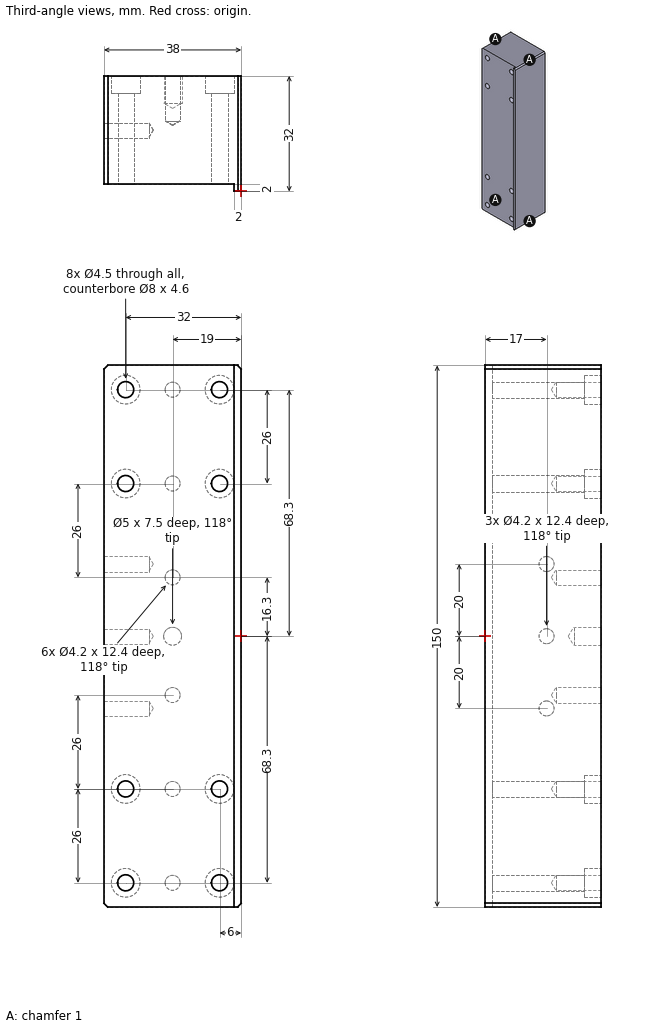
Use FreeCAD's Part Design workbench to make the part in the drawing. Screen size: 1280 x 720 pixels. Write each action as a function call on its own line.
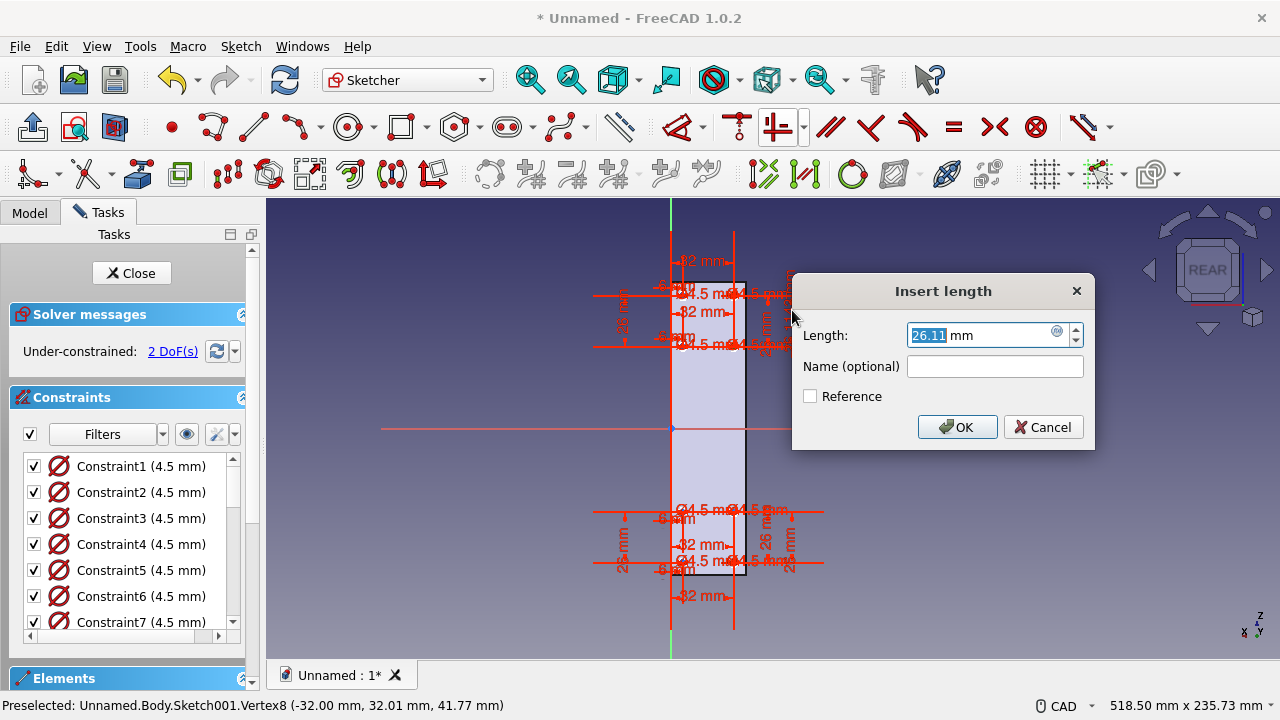
text(26)
key(Return)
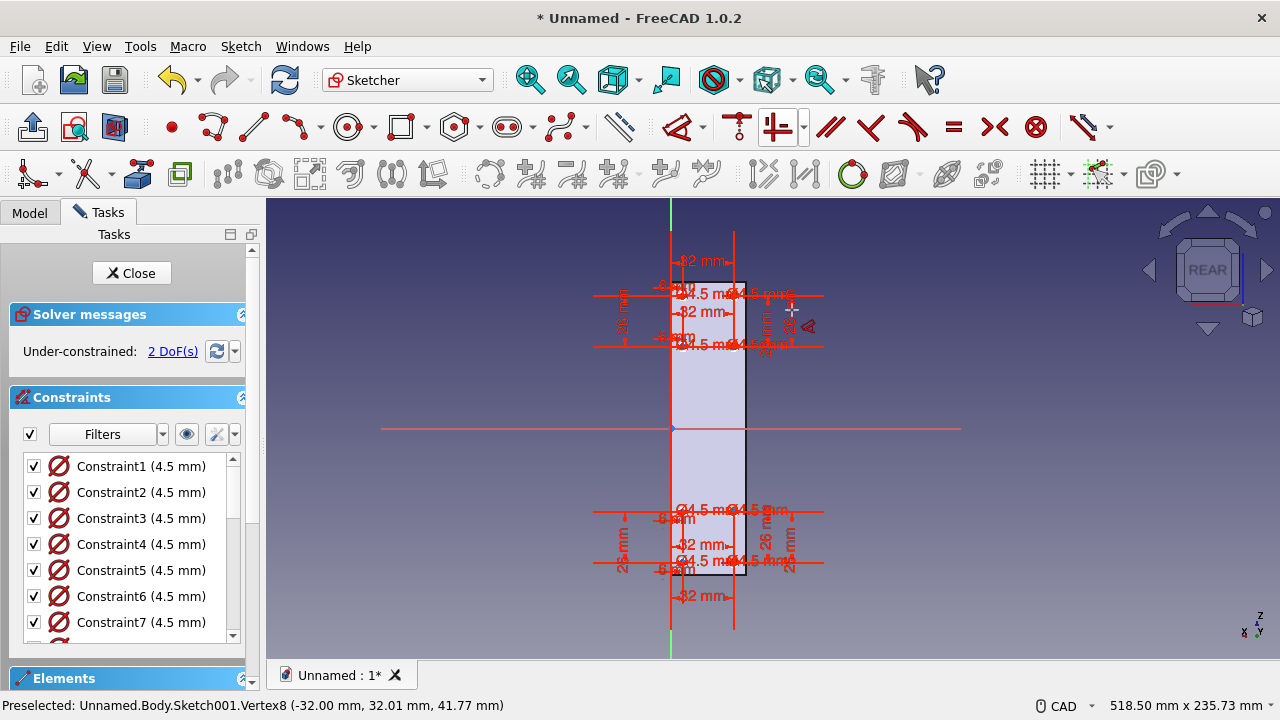
click(734, 296)
click(637, 362)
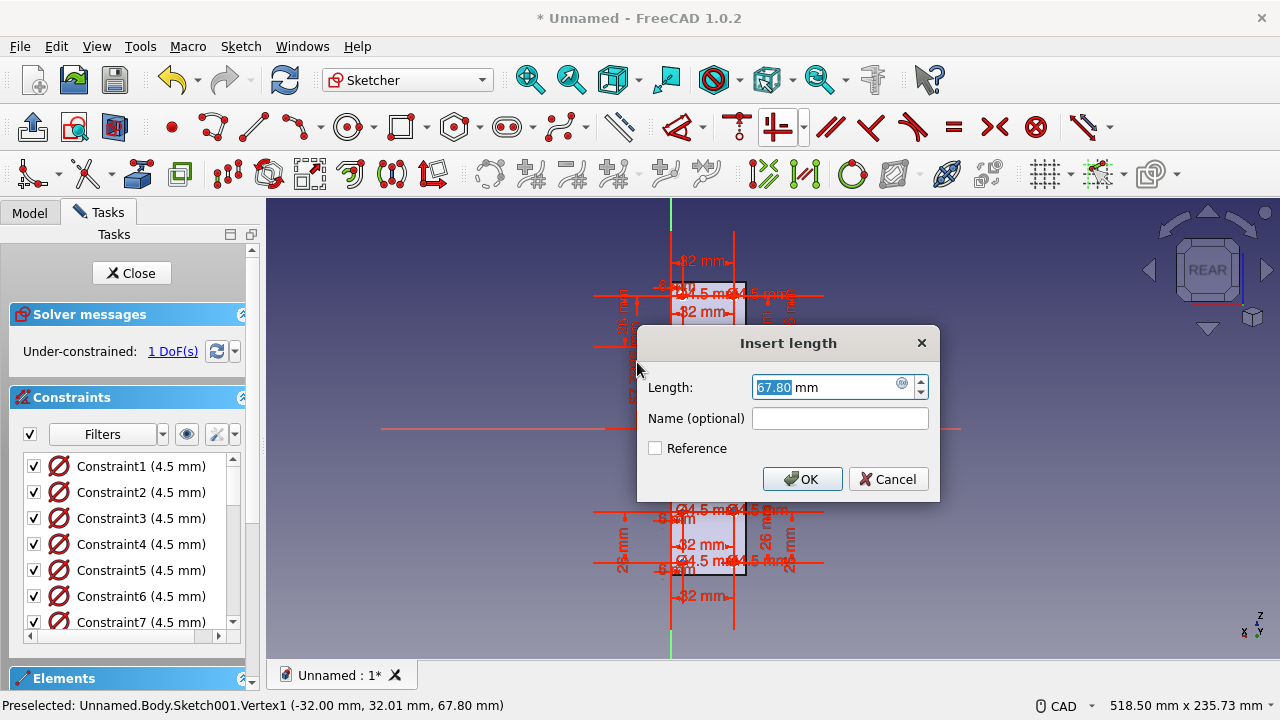
text(68.3)
key(Return)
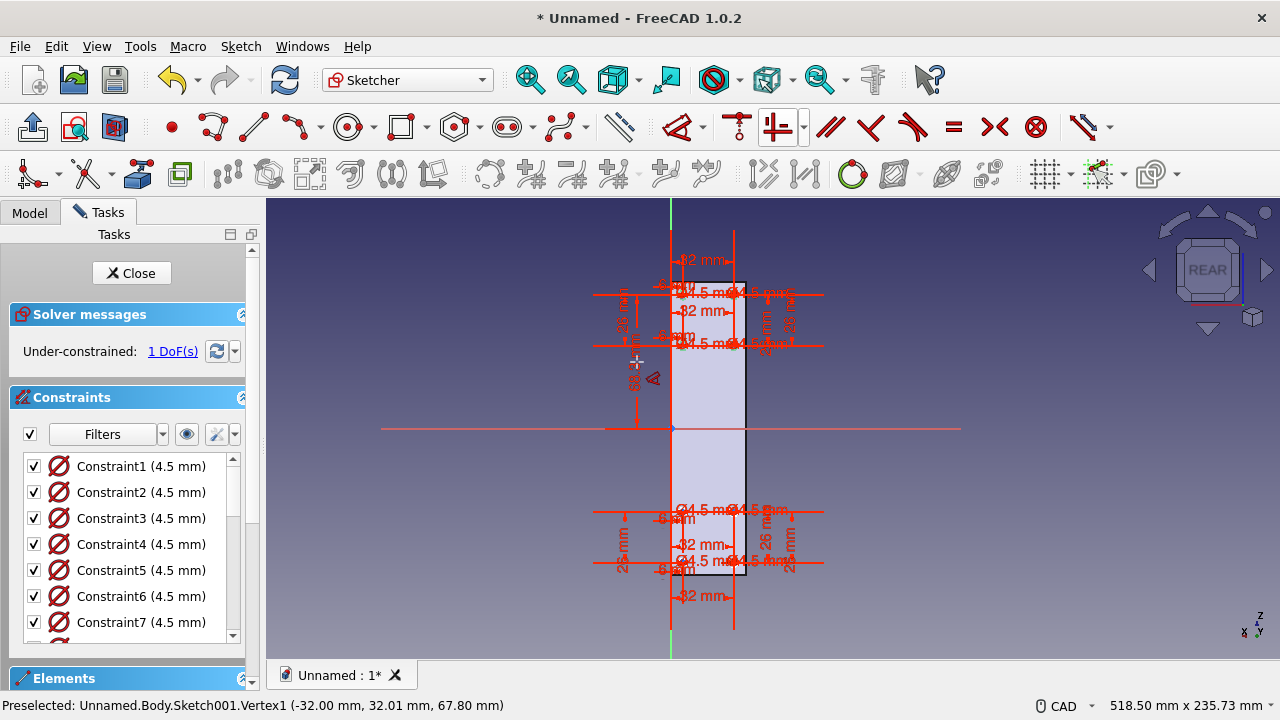
click(734, 563)
click(637, 496)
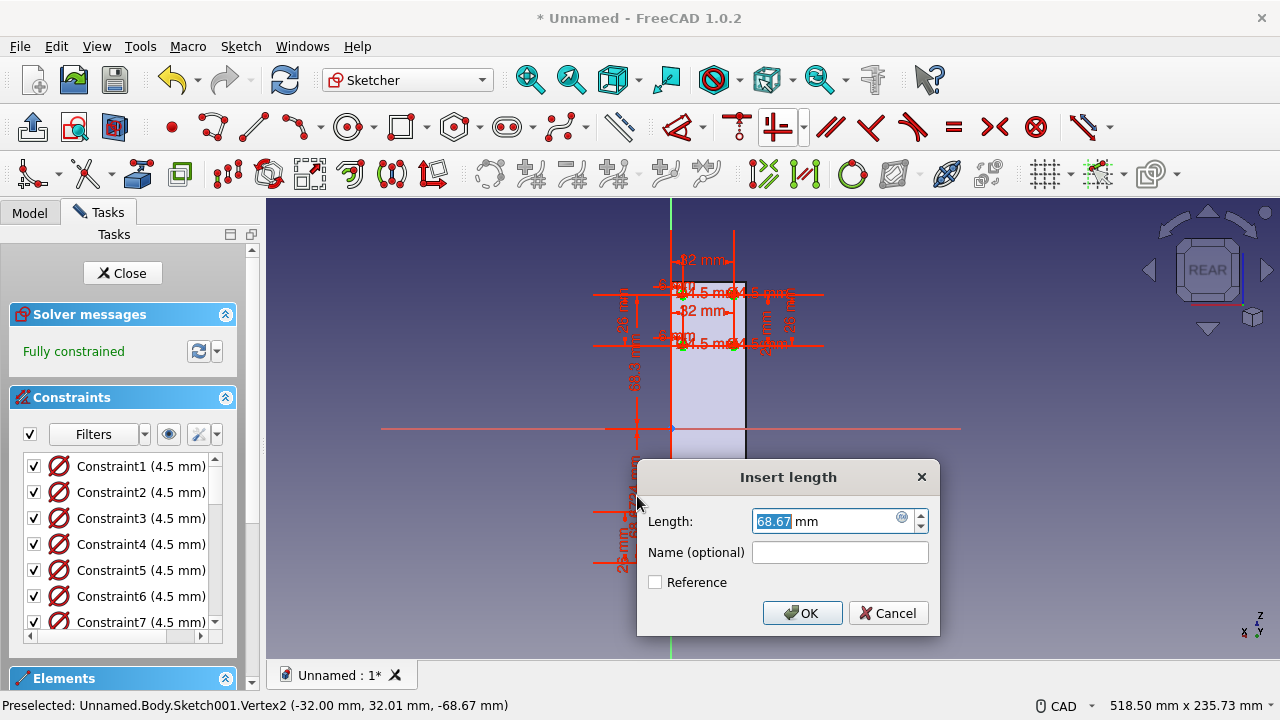
text(68.3)
key(Return)
key(Escape)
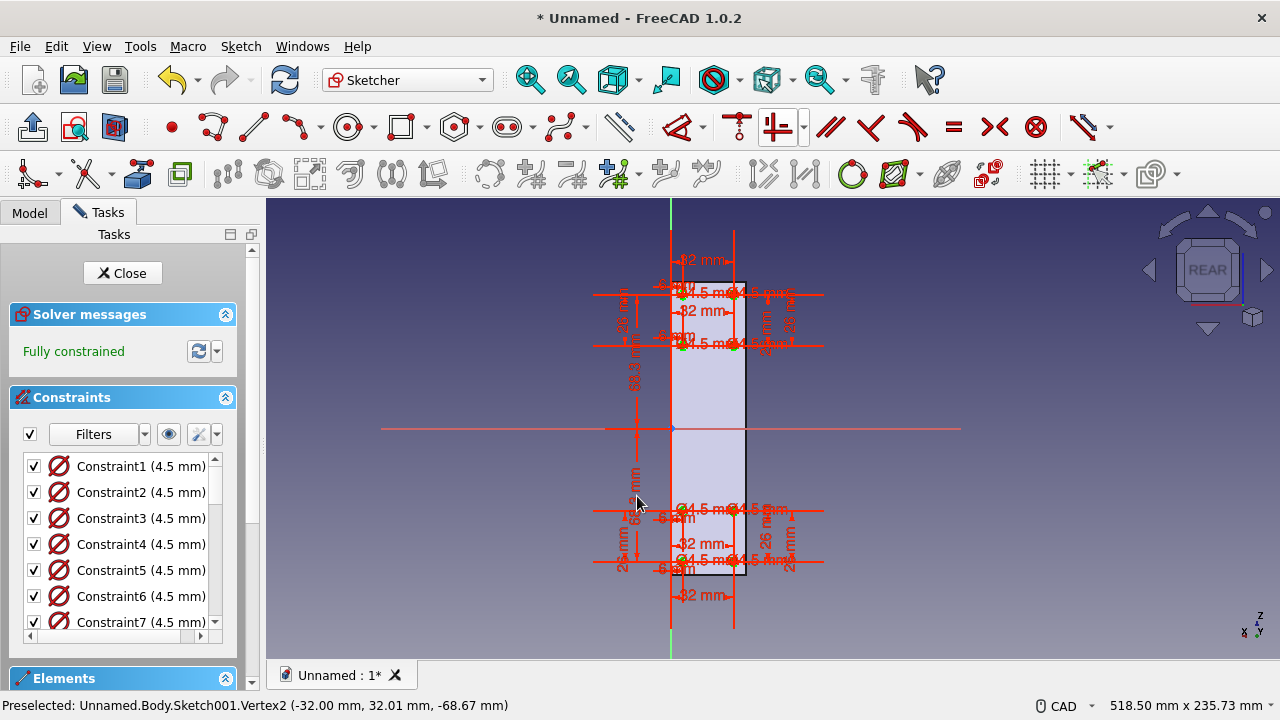
click(123, 273)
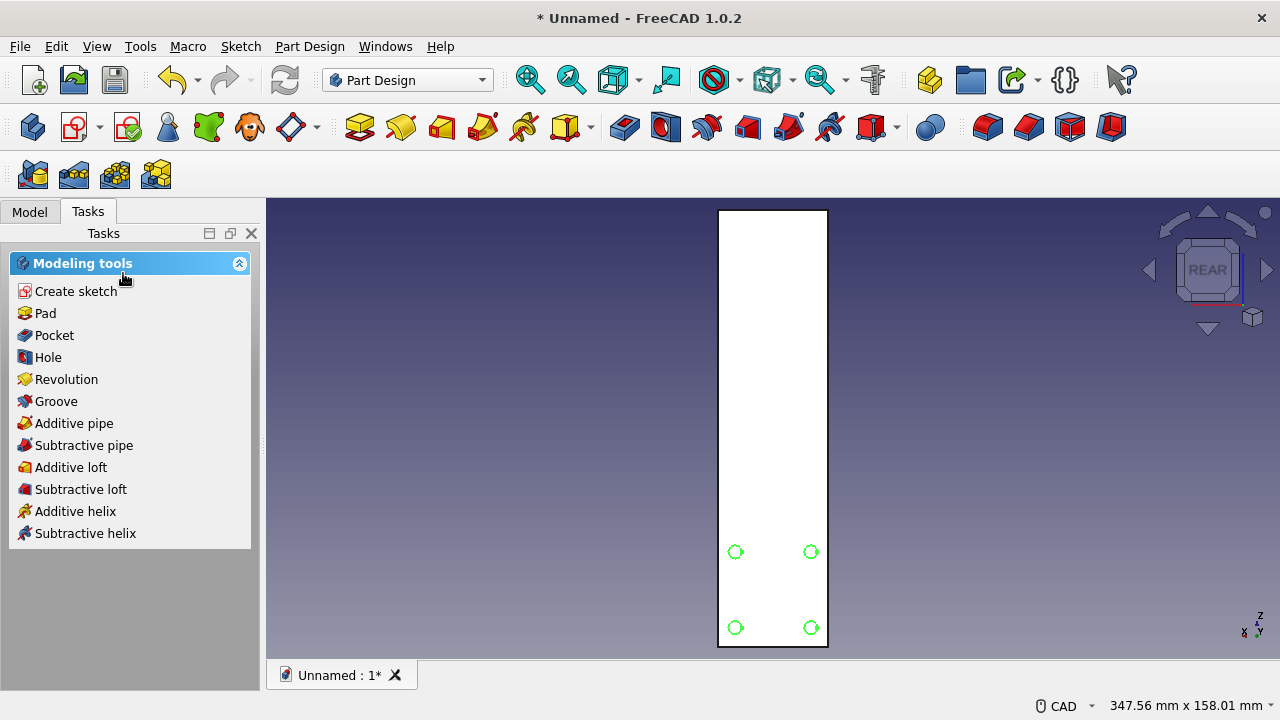
click(666, 128)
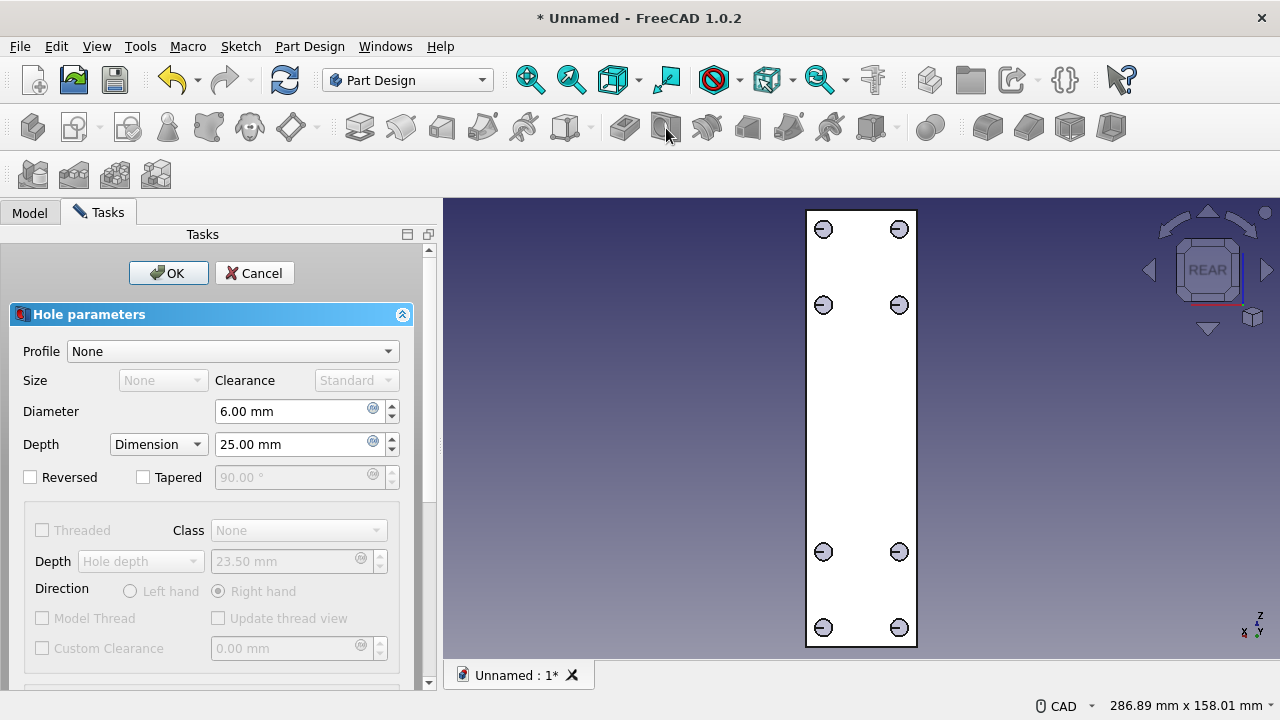
triple_click(300, 412)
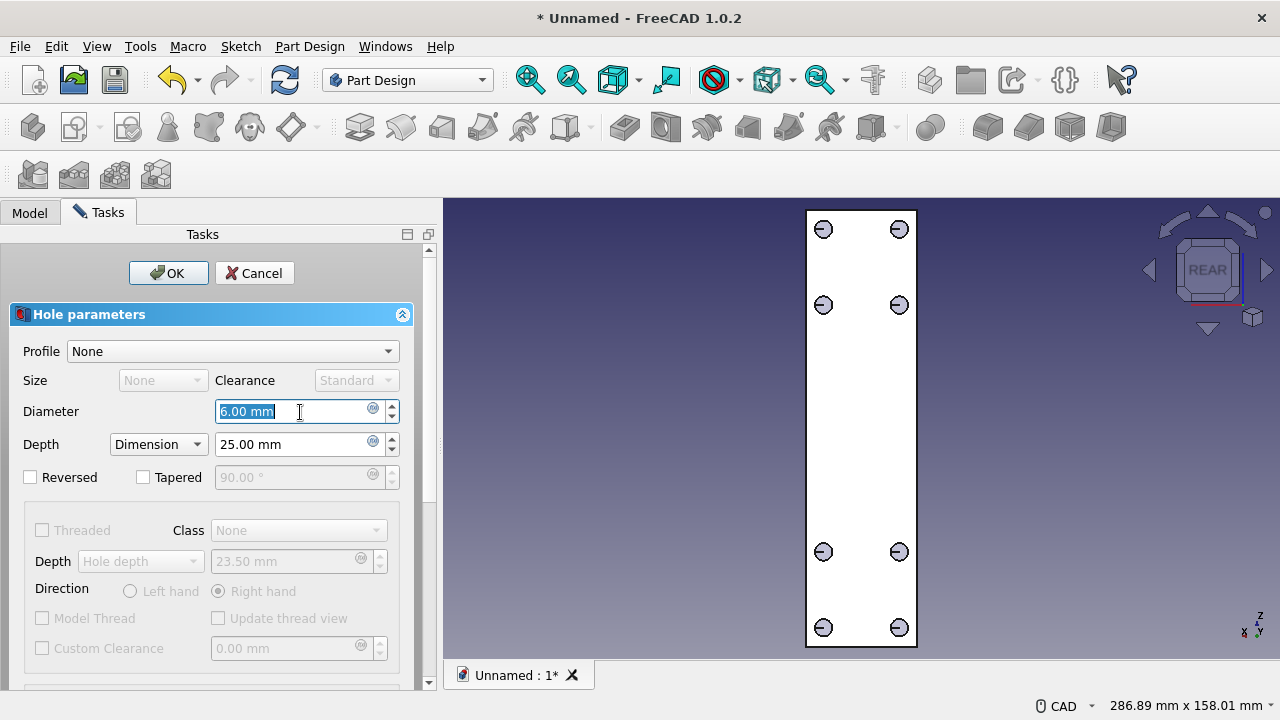
text(4.5)
key(Tab)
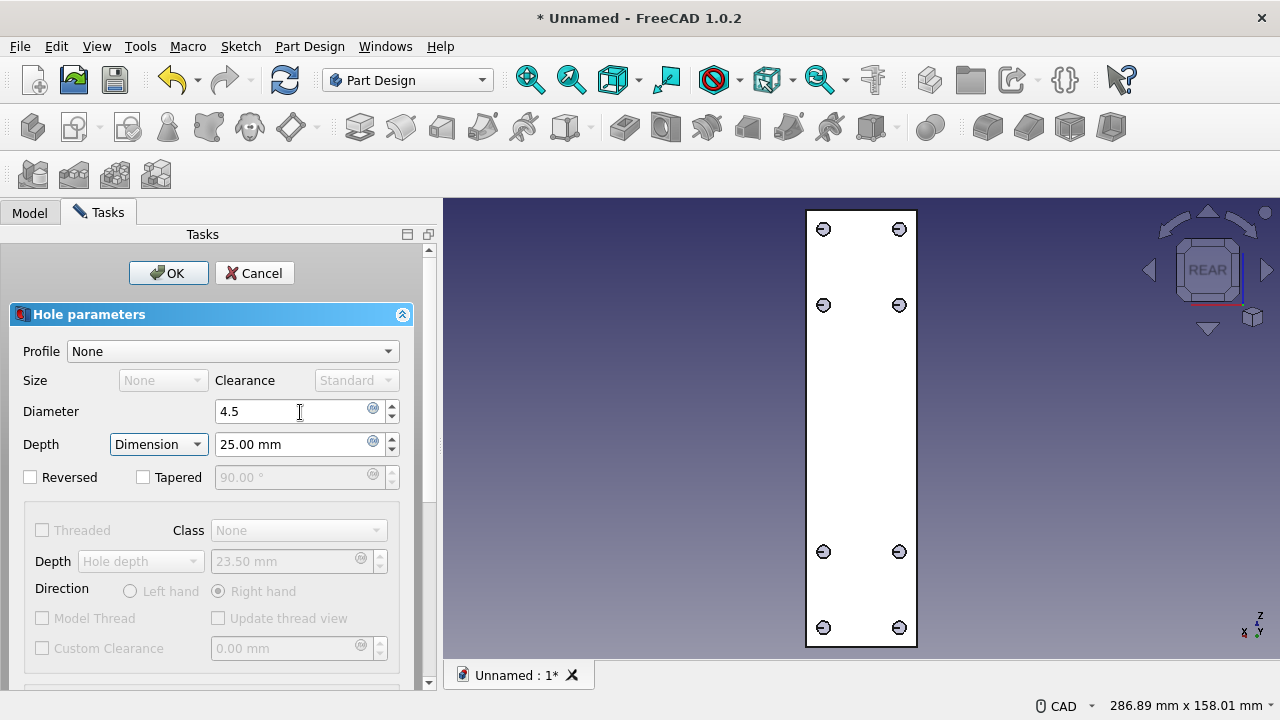
click(160, 444)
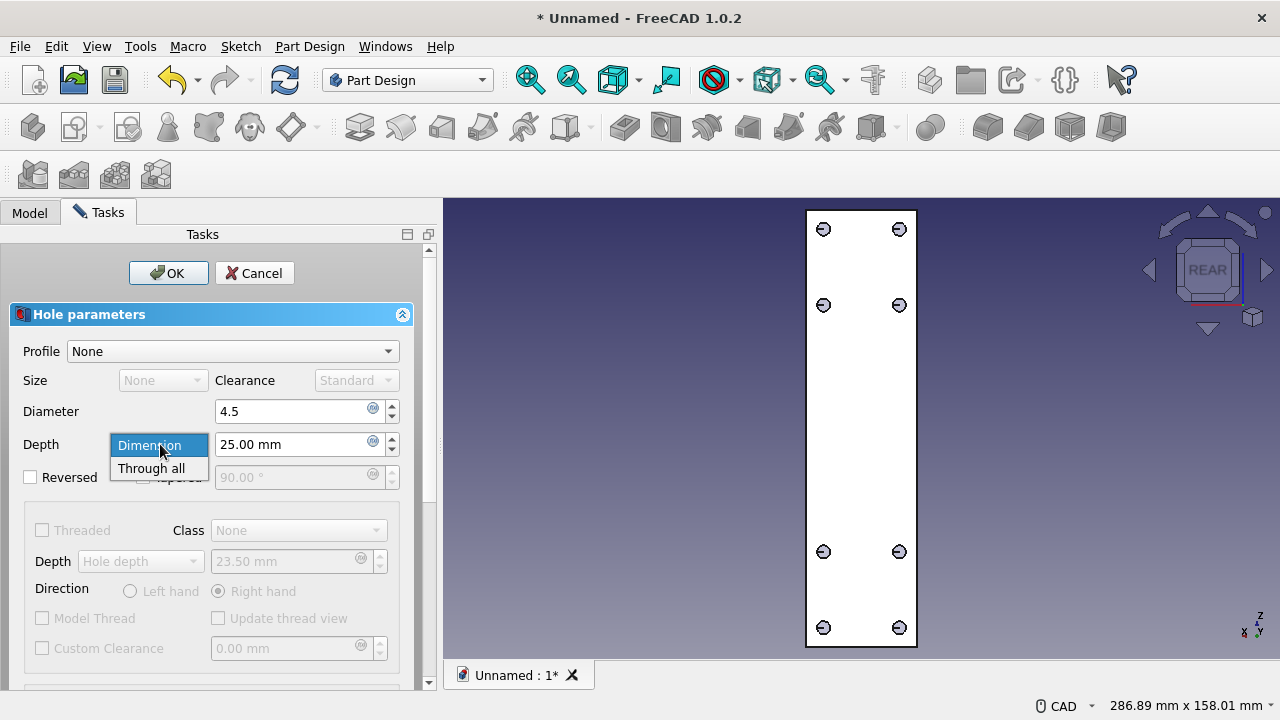
click(158, 468)